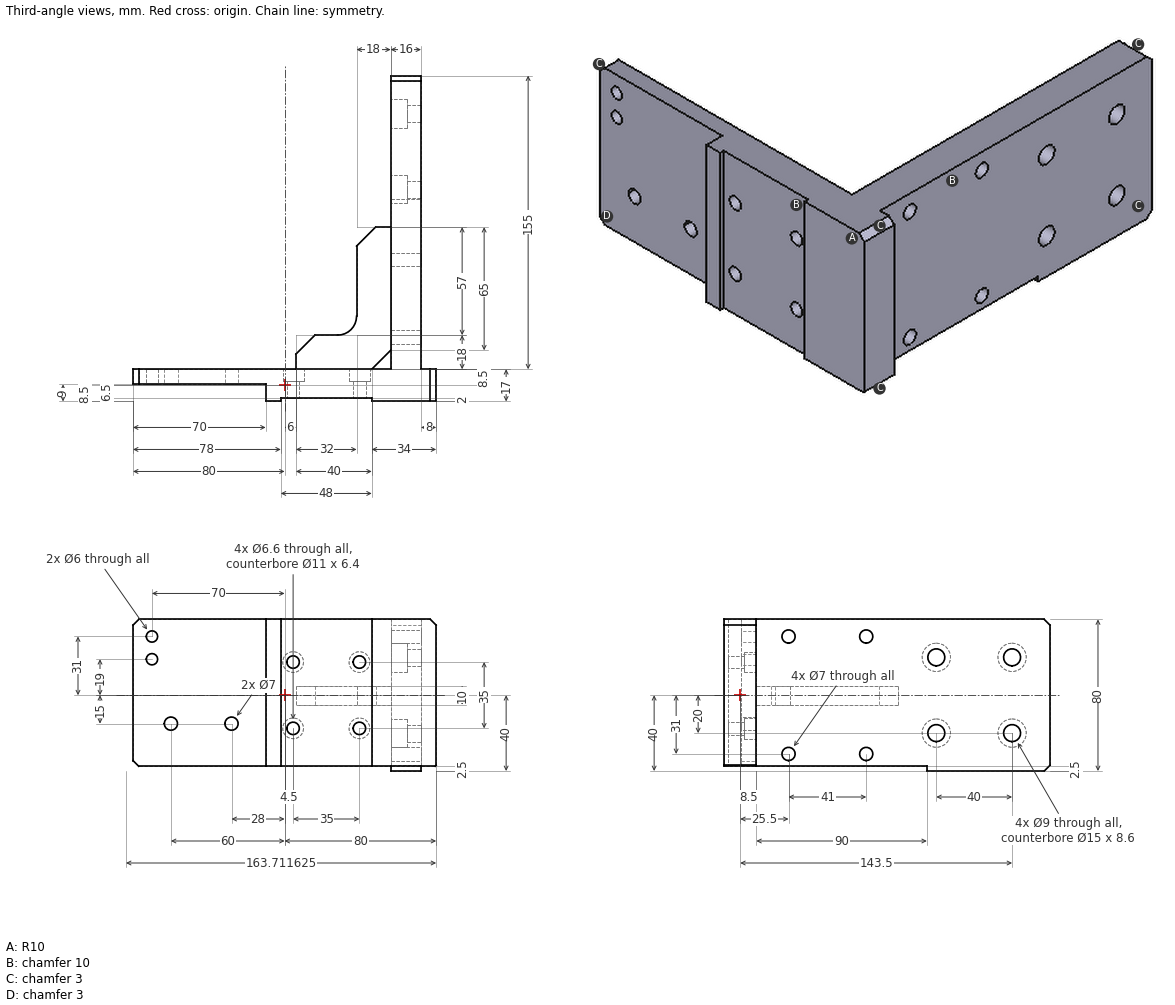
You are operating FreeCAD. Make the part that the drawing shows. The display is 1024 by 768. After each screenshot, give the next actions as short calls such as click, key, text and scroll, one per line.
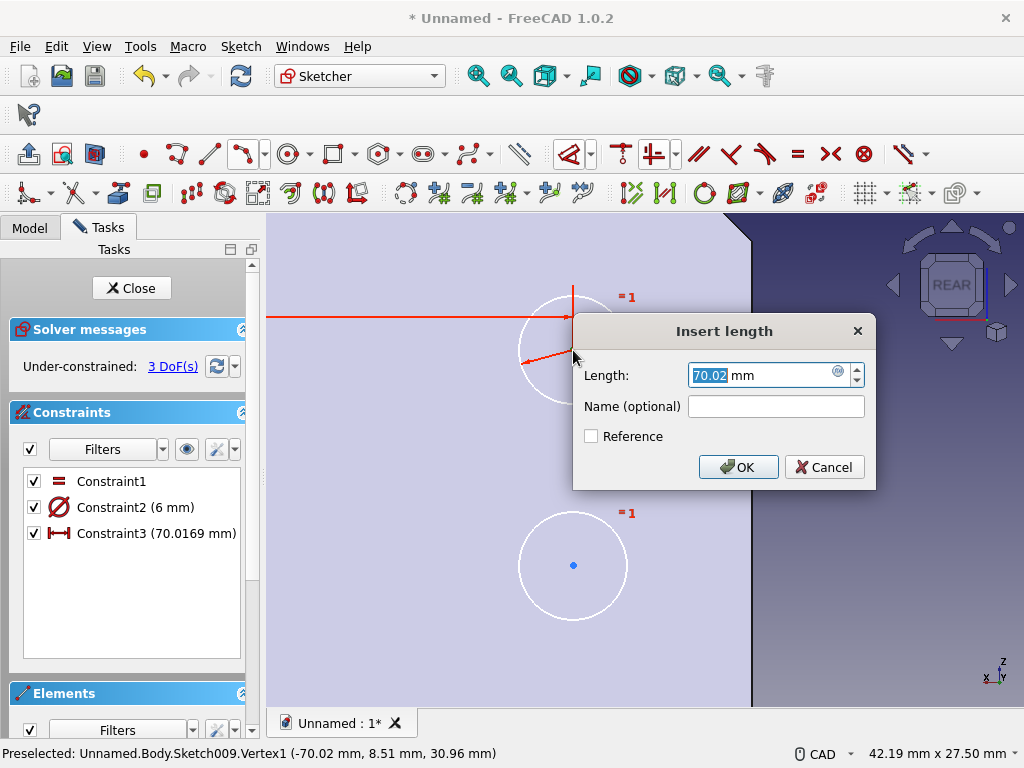
text(70)
key(Return)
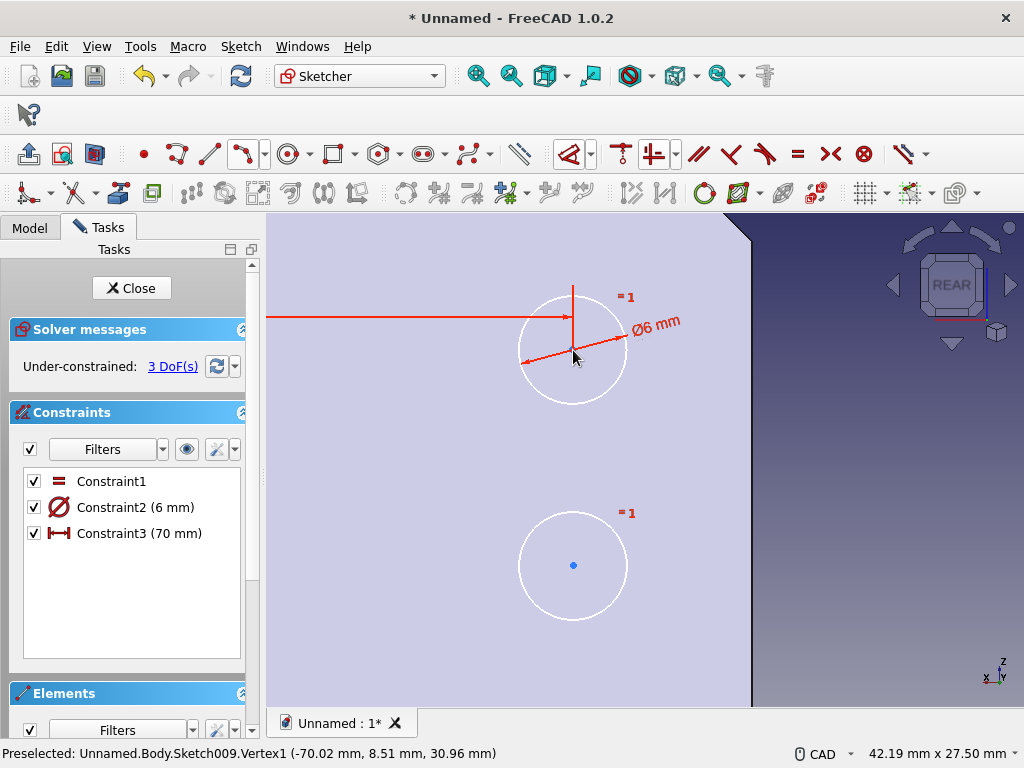
click(573, 350)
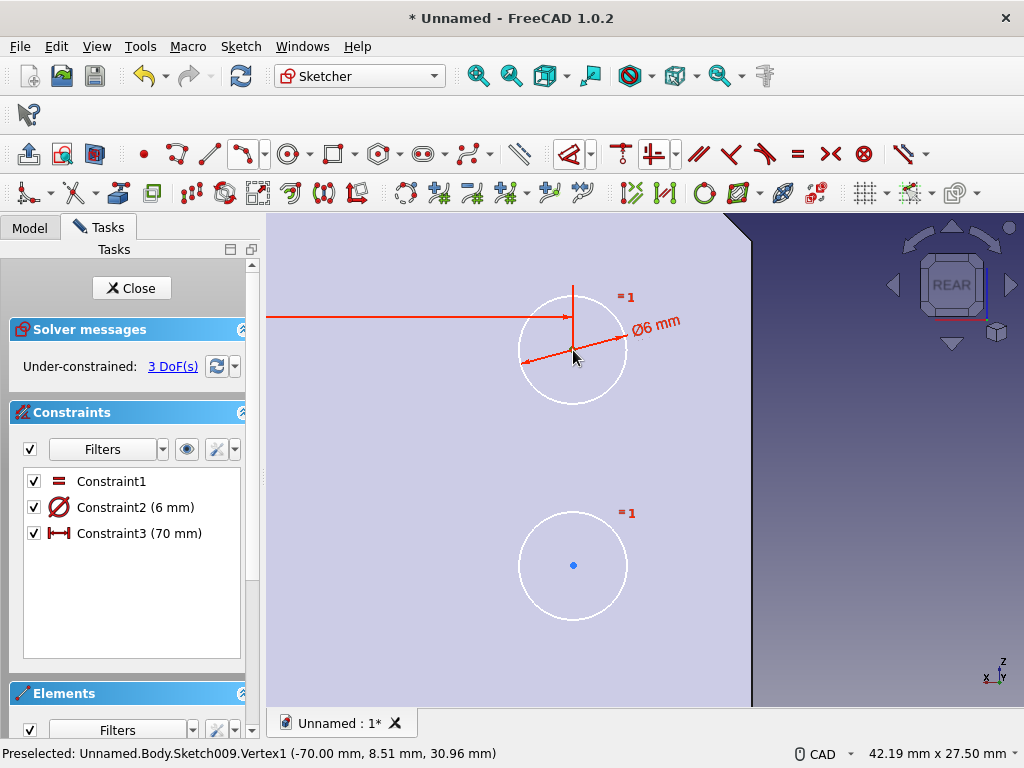
click(590, 154)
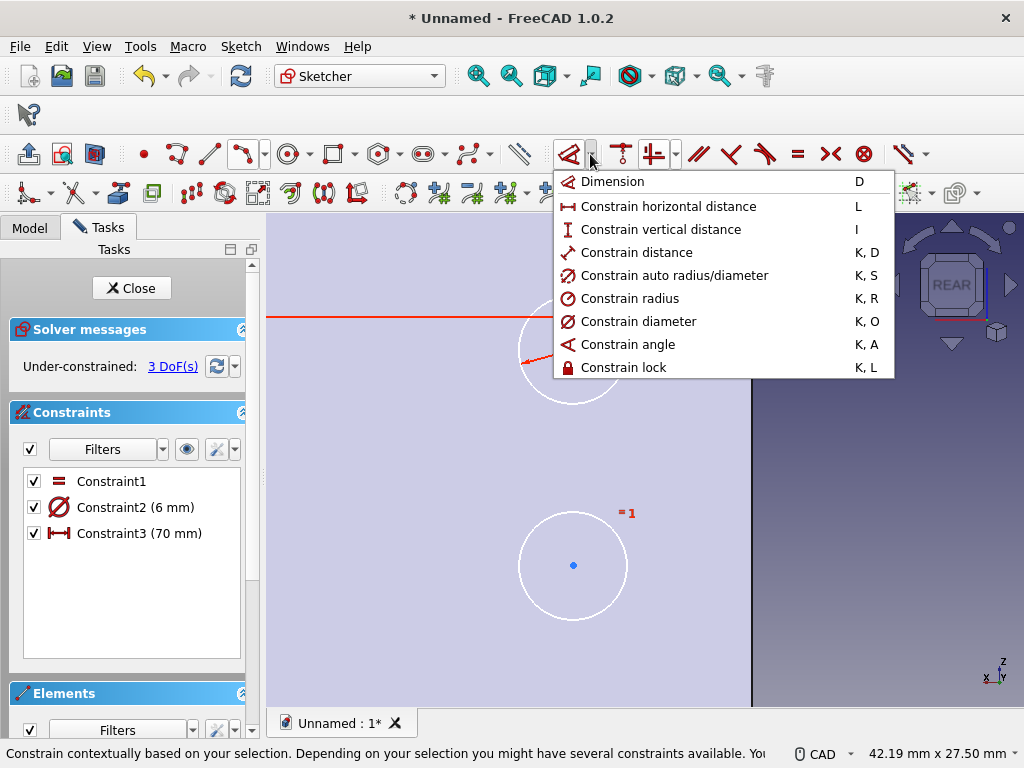
click(724, 230)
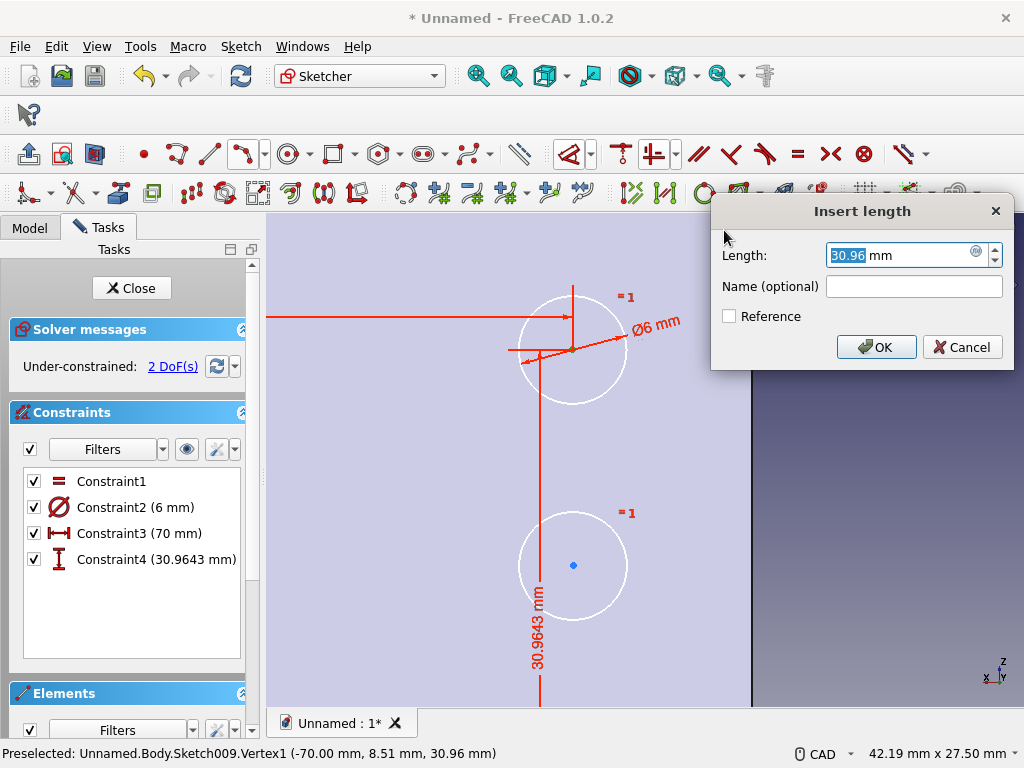
text(31)
key(Return)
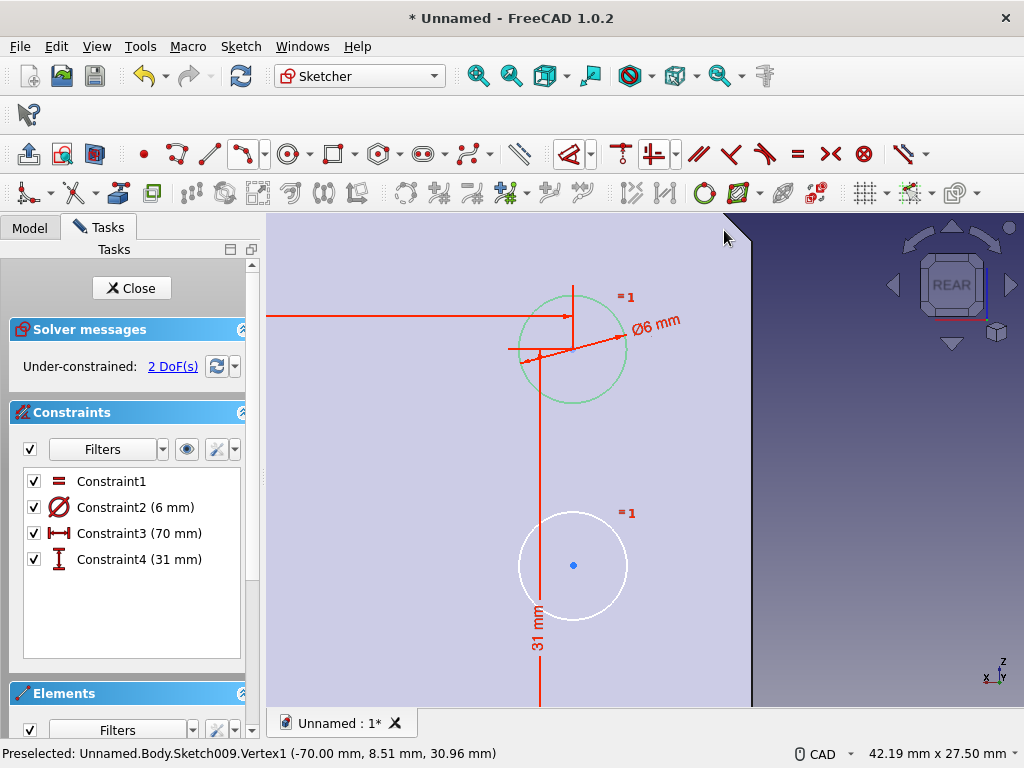
click(573, 566)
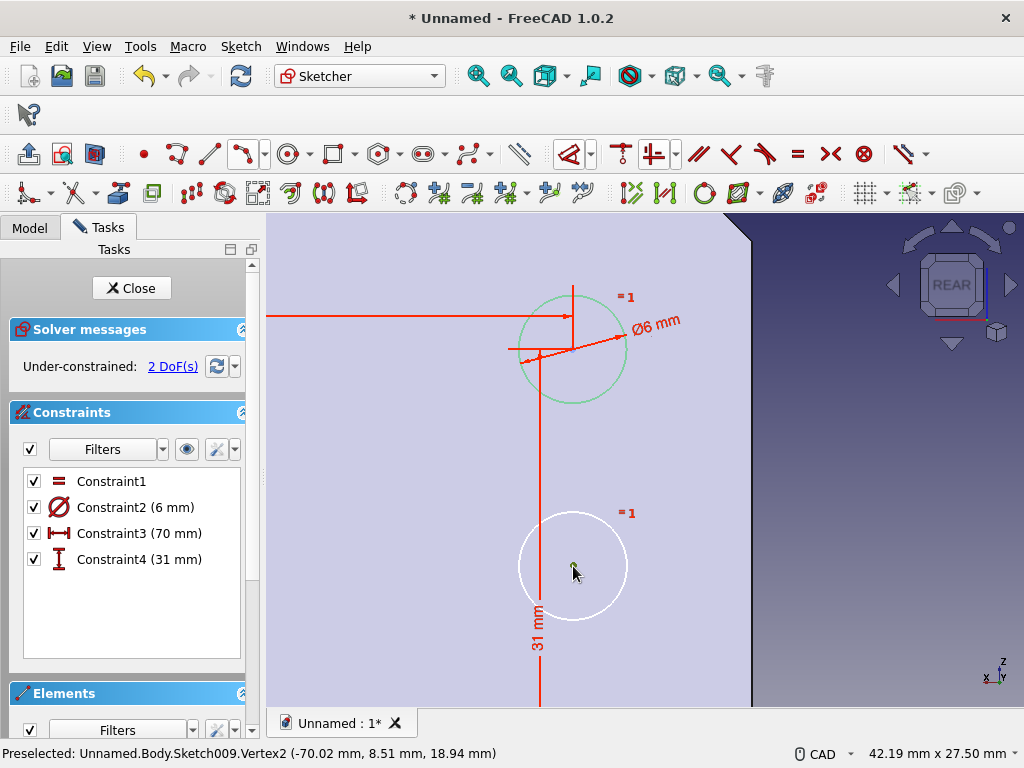
click(590, 154)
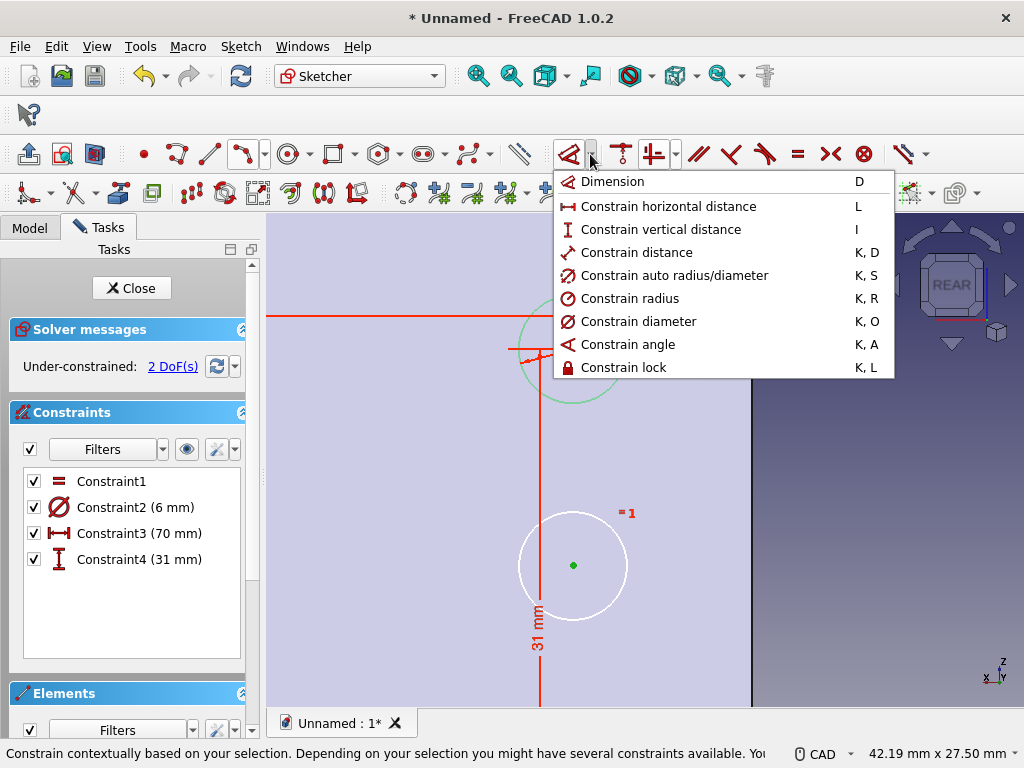
click(724, 206)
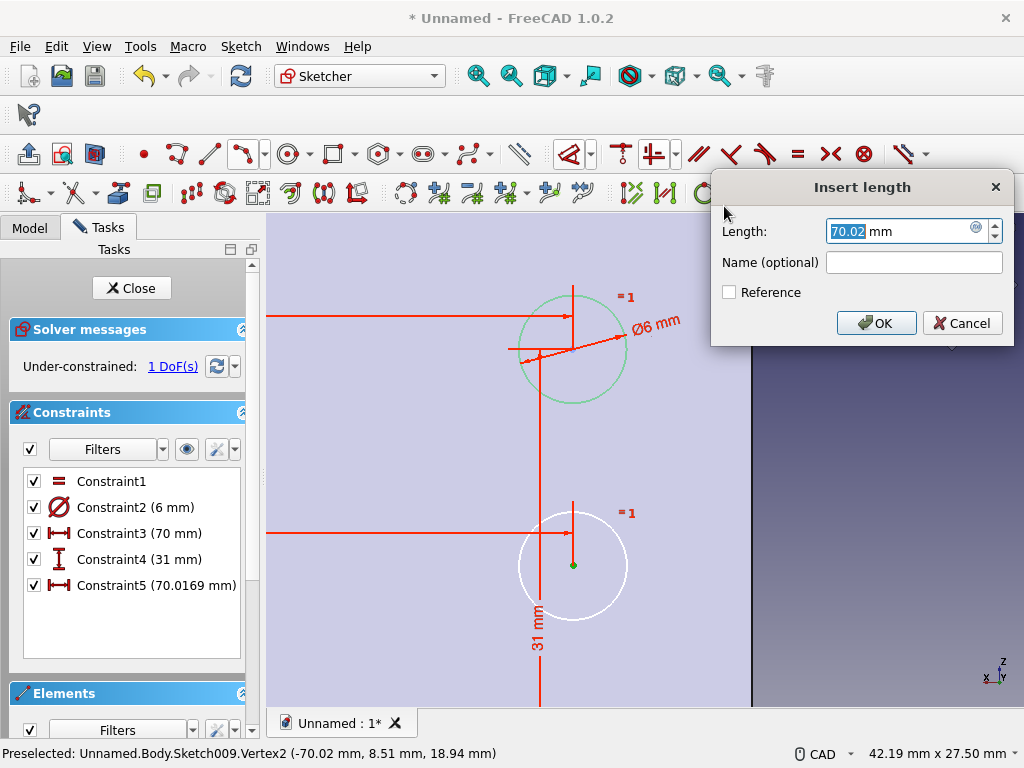
text(70)
key(Return)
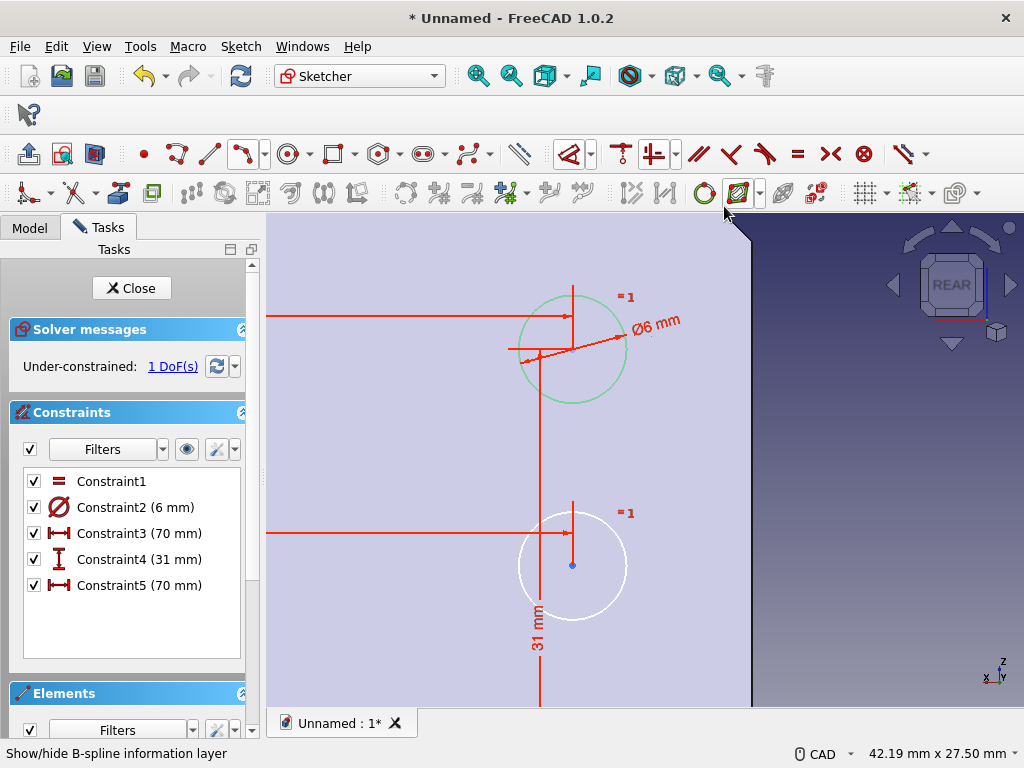
click(573, 566)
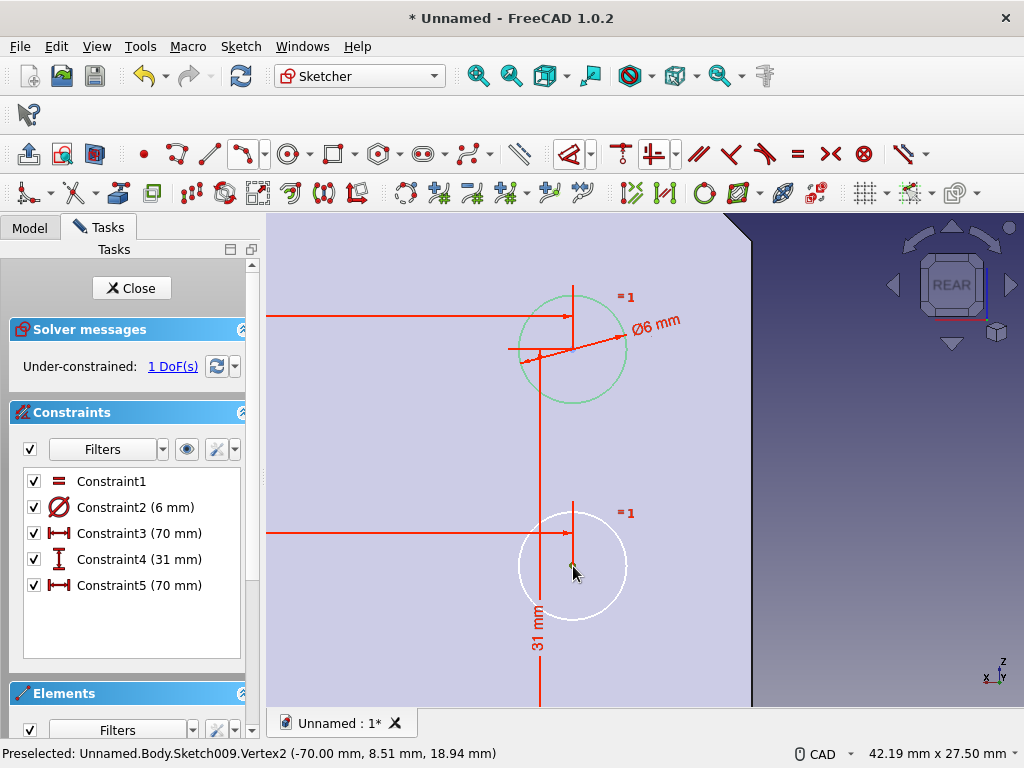
click(590, 154)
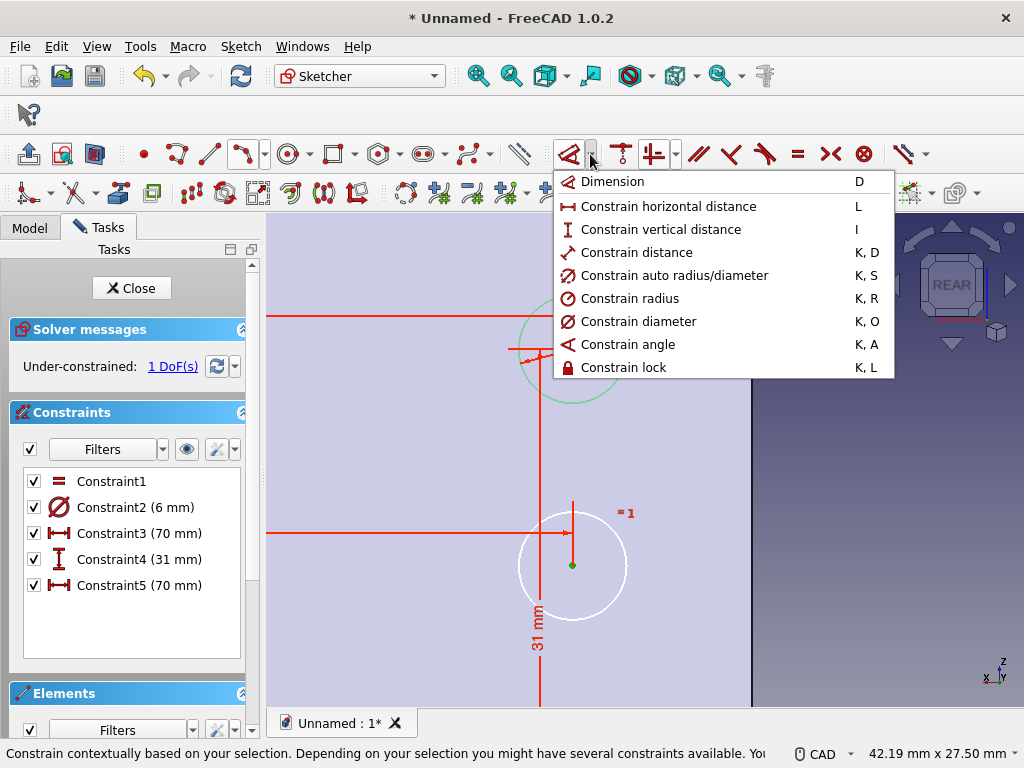
click(724, 230)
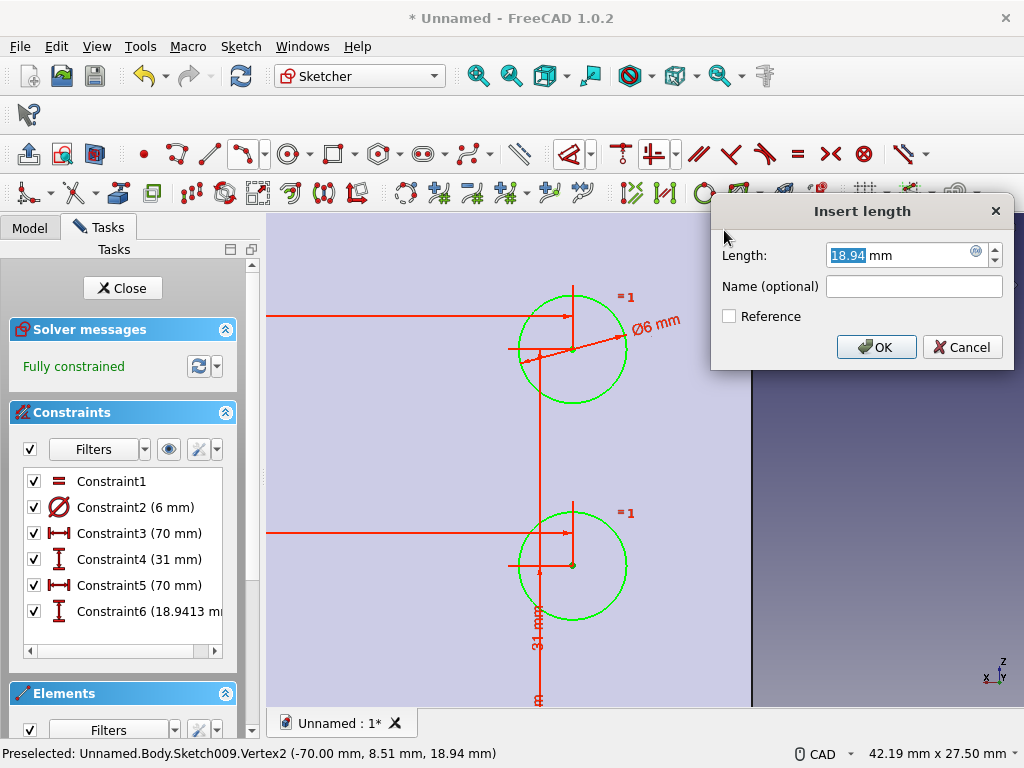
text(19)
key(Return)